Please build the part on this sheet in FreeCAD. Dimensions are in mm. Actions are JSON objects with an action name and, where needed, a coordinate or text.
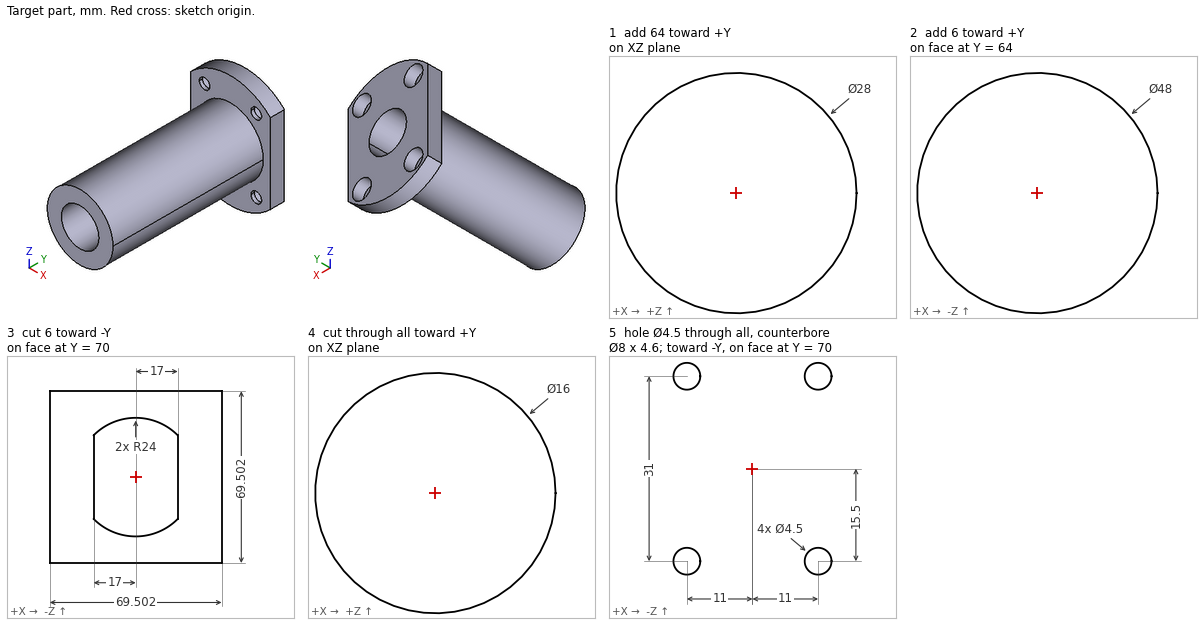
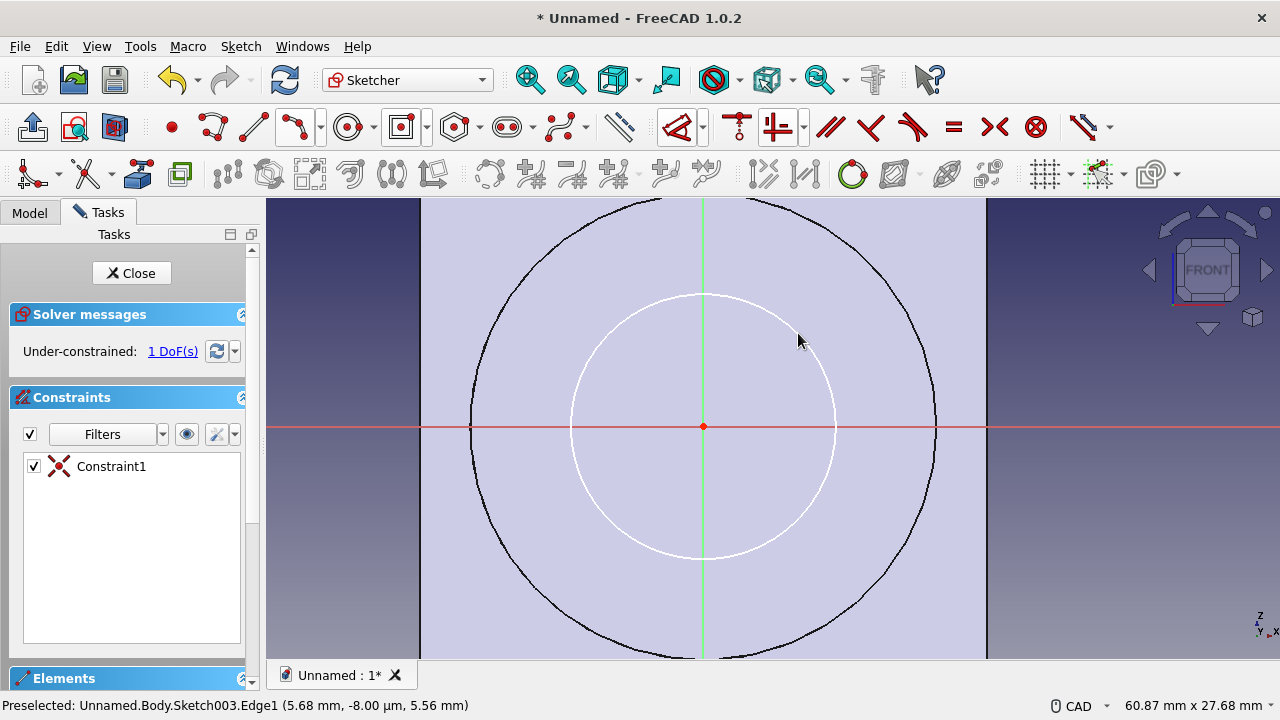
{"action": "left_click", "coordinate": [797, 333]}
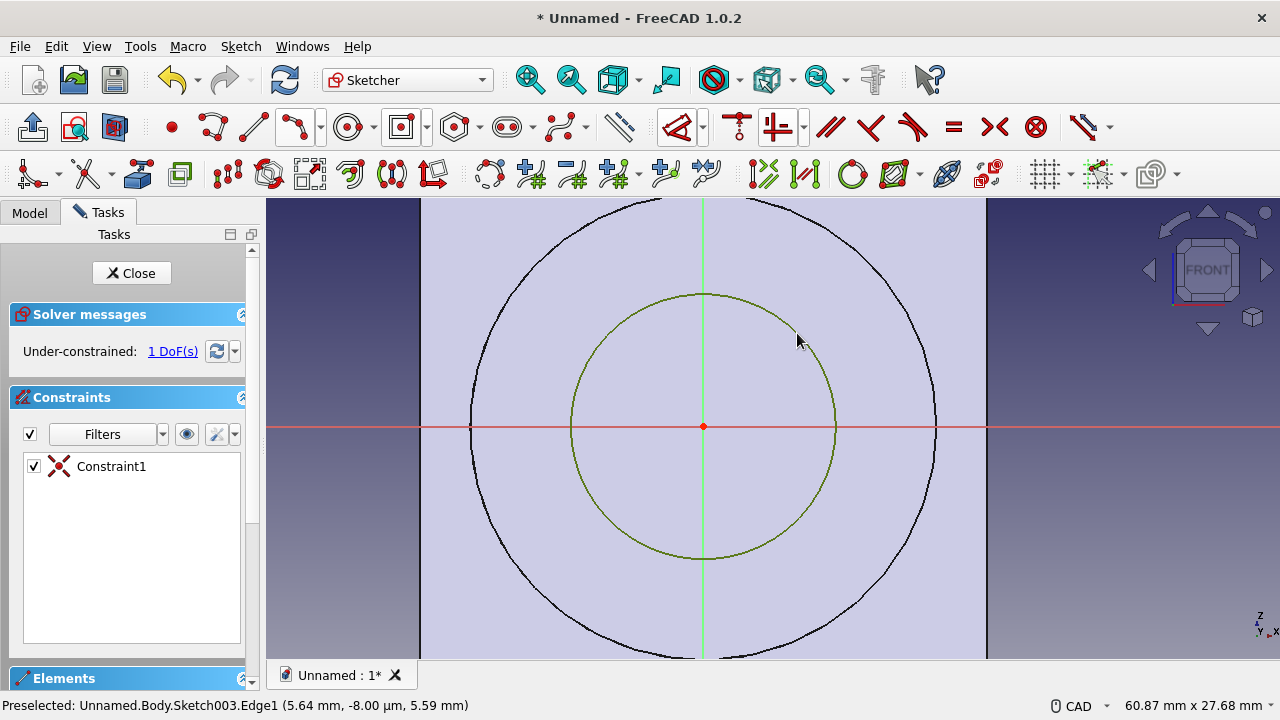
{"action": "left_click", "coordinate": [702, 128]}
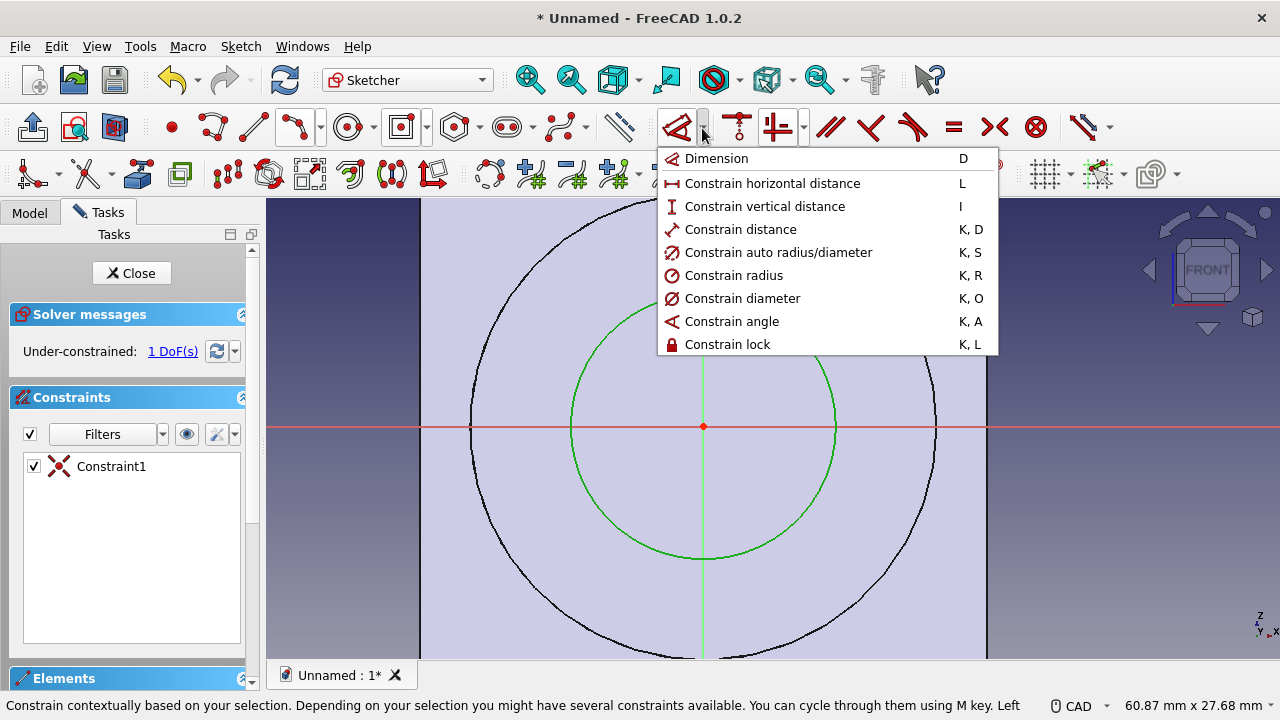
{"action": "left_click", "coordinate": [828, 298]}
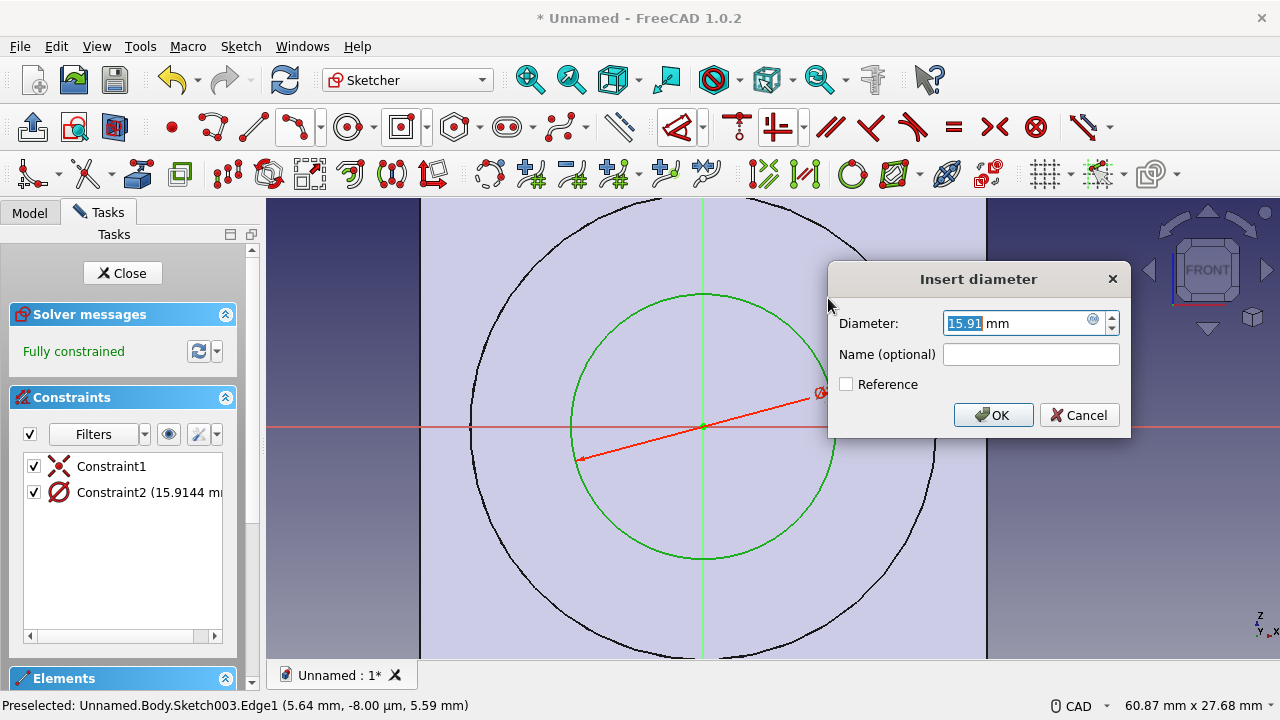
{"action": "type", "text": "16"}
{"action": "key", "text": "Return"}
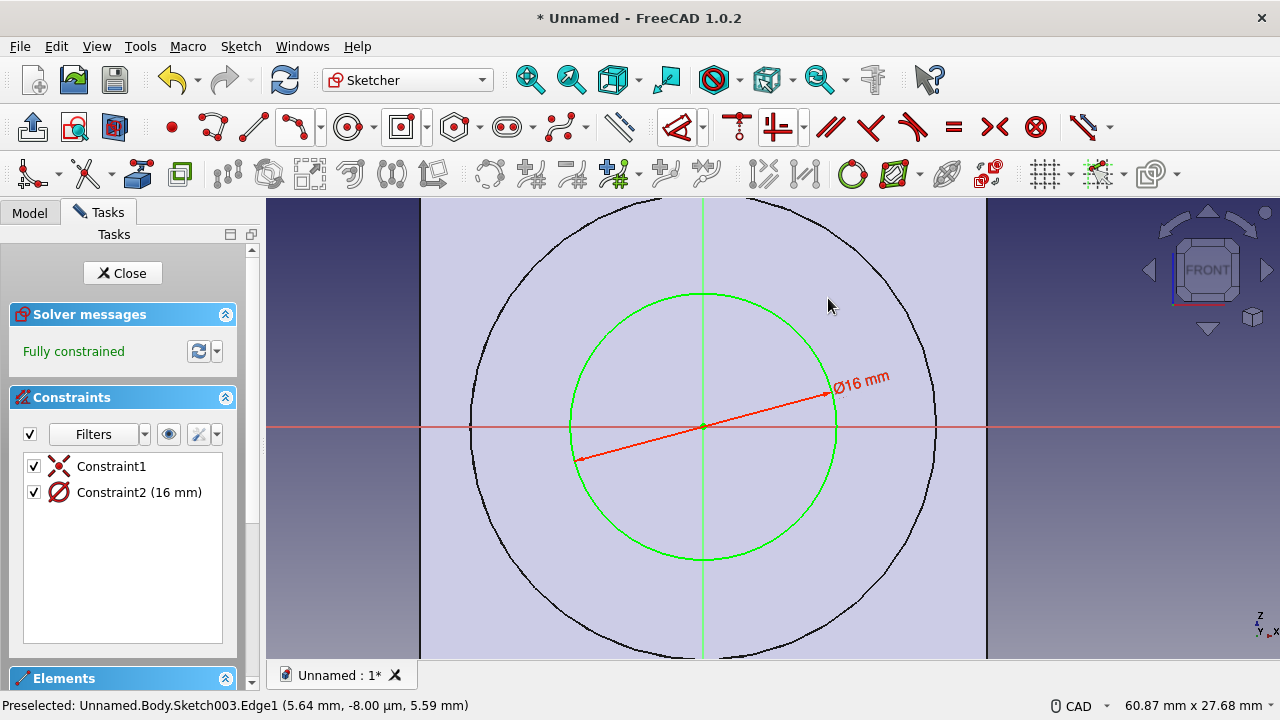
{"action": "left_click", "coordinate": [123, 273]}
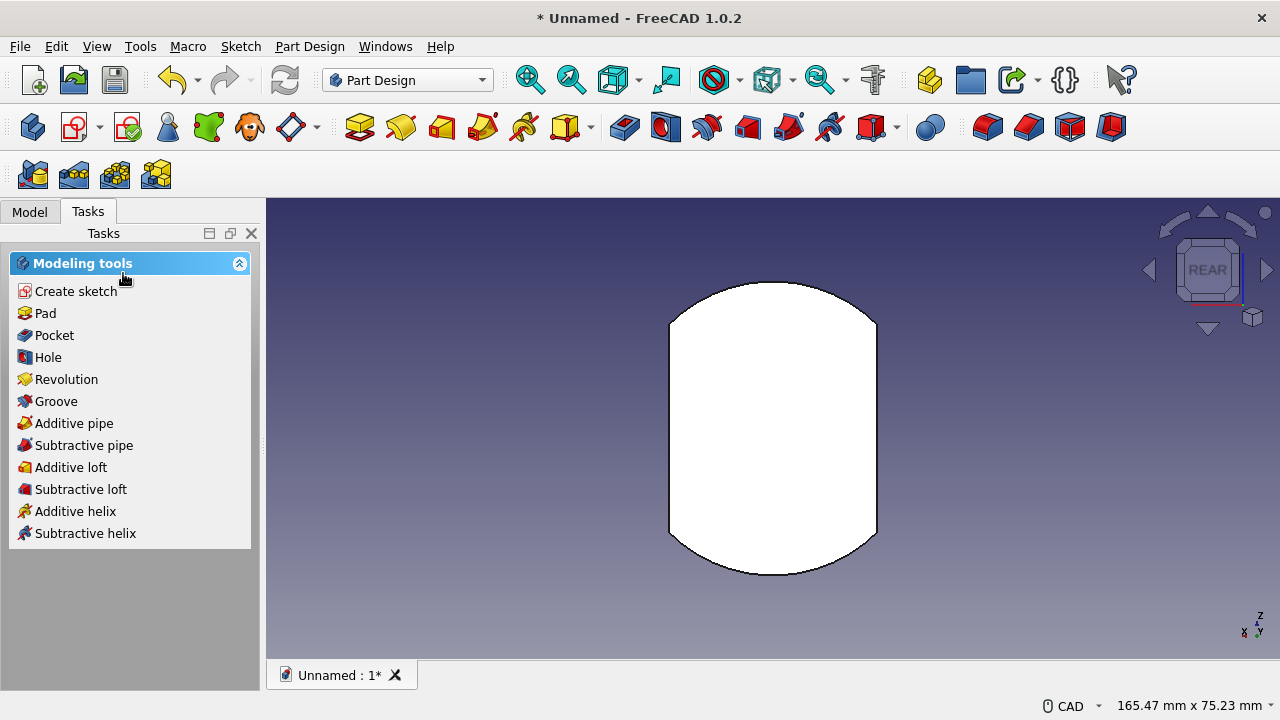
{"action": "left_click", "coordinate": [625, 128]}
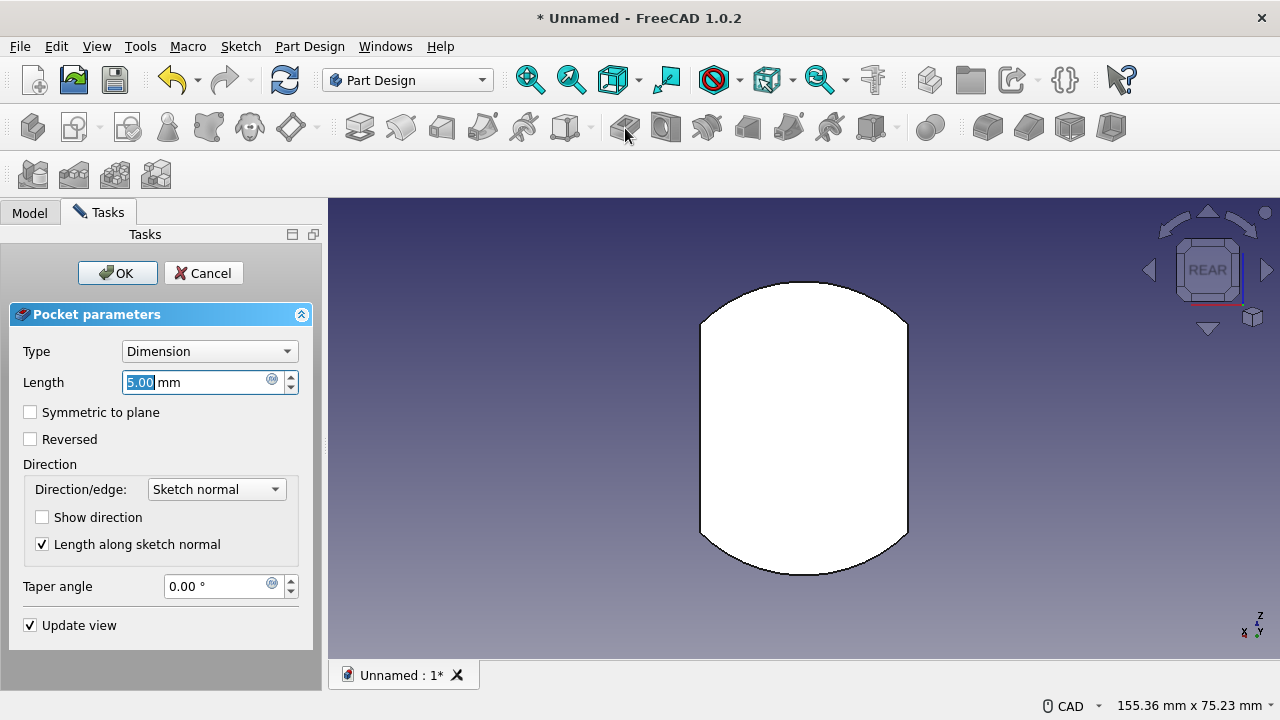
{"action": "left_click", "coordinate": [210, 352]}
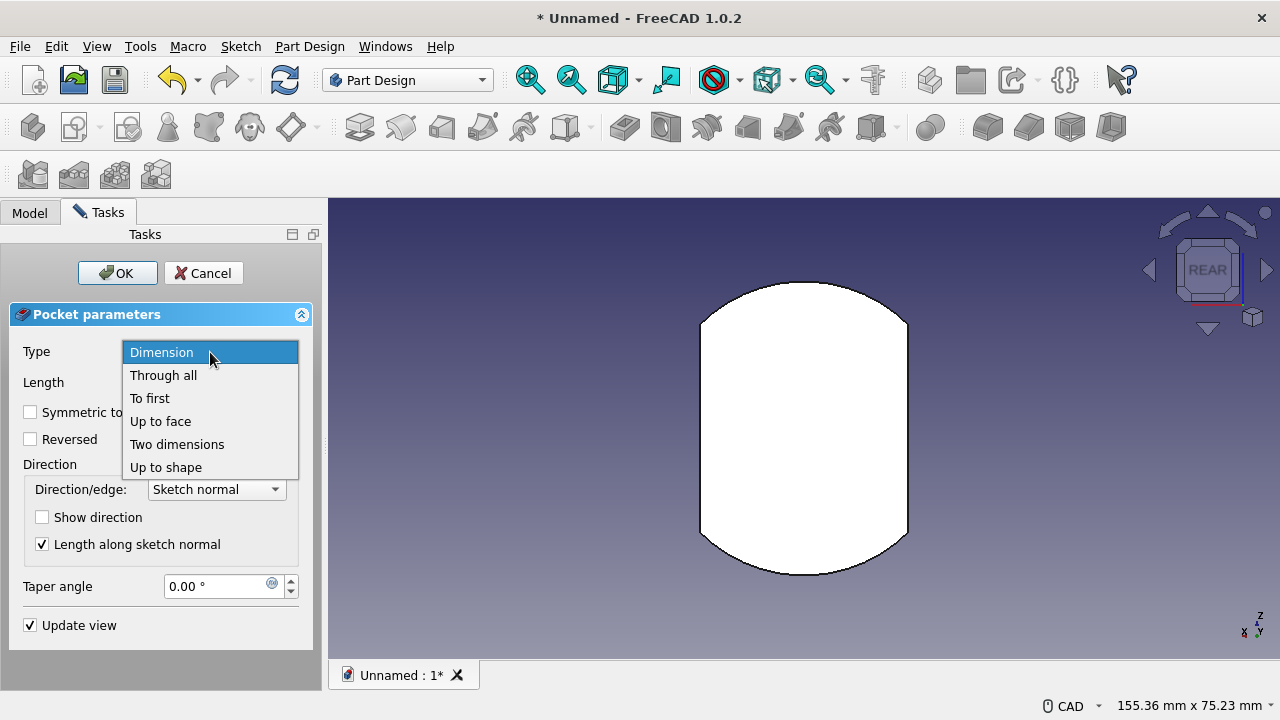
{"action": "left_click", "coordinate": [208, 376]}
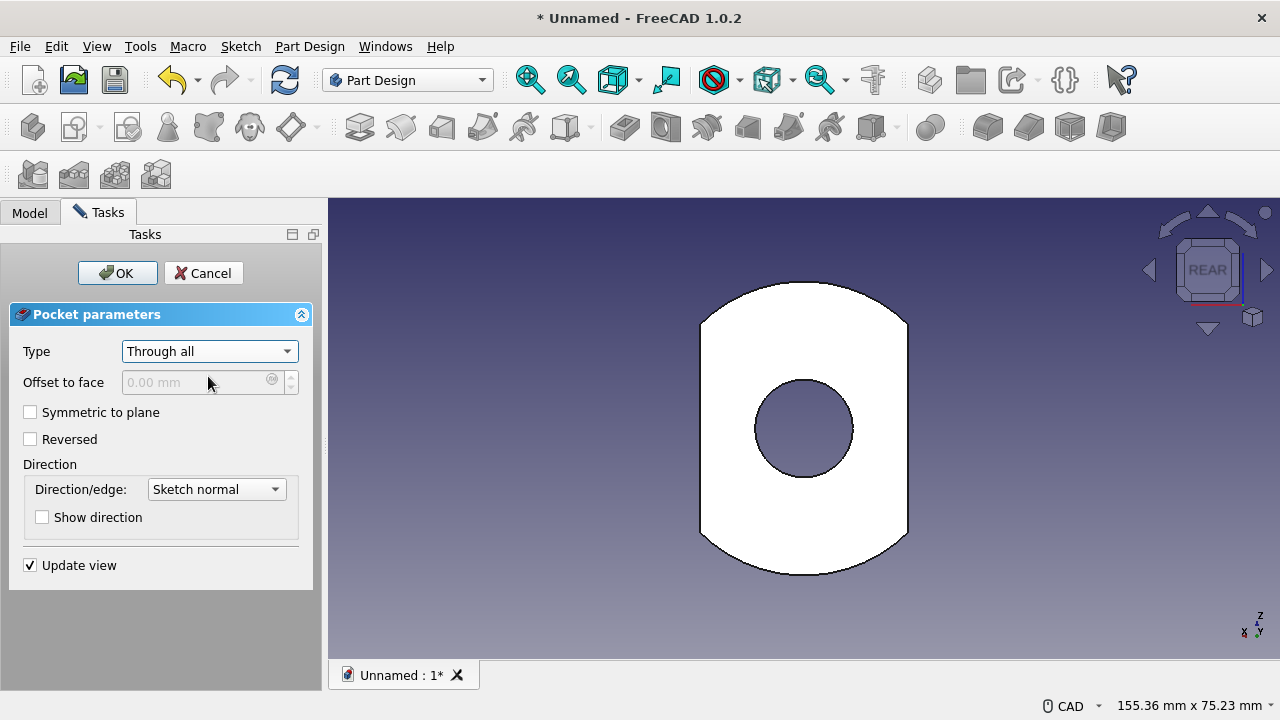
{"action": "left_click", "coordinate": [118, 273]}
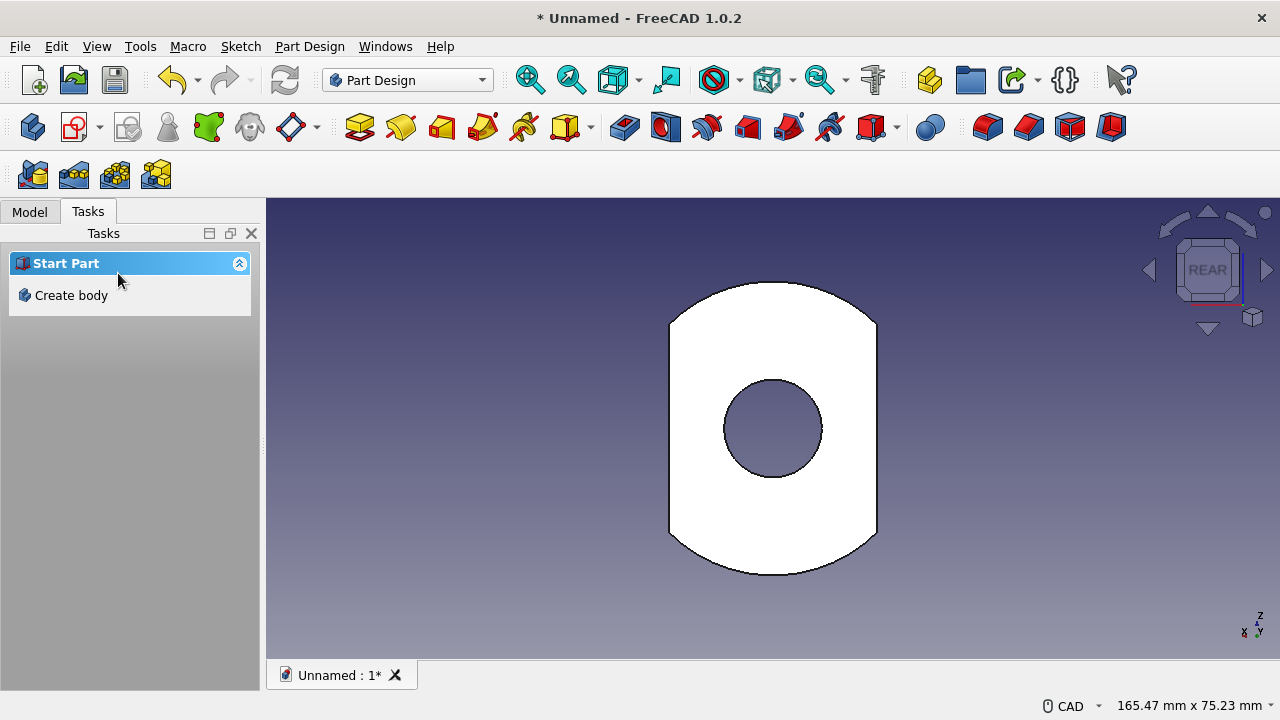
{"action": "left_click", "coordinate": [713, 512]}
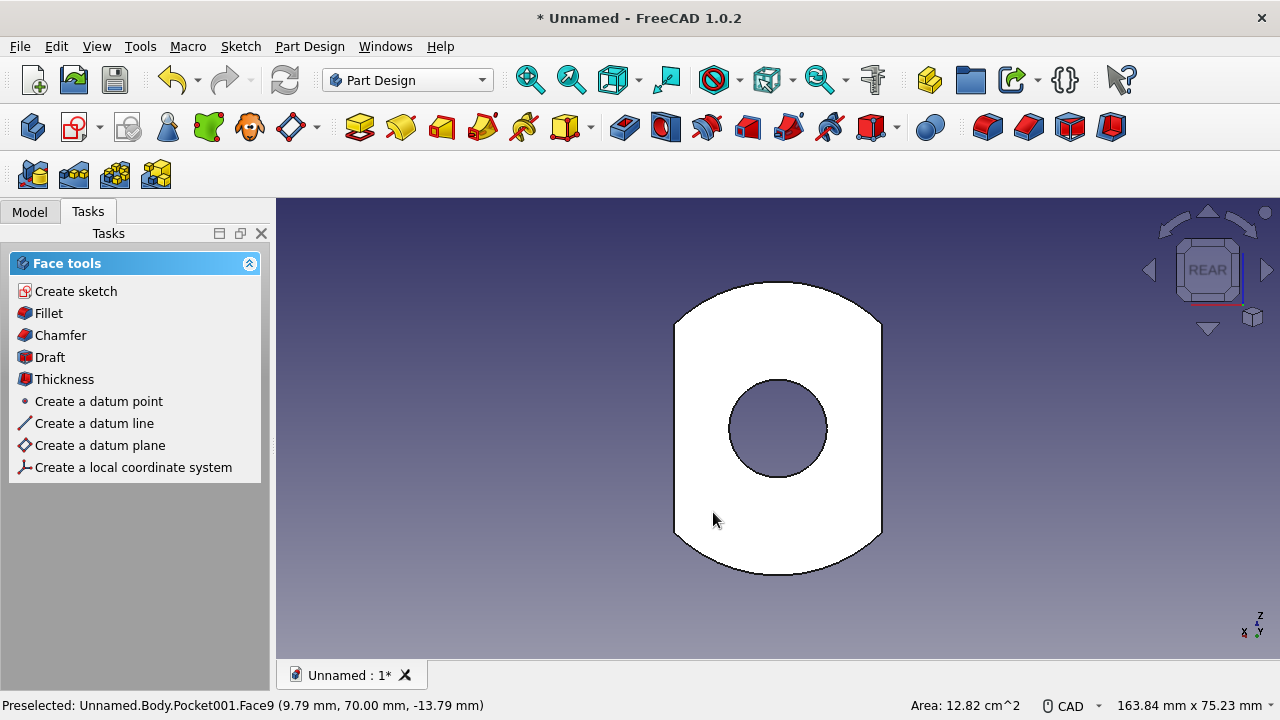
{"action": "left_click", "coordinate": [74, 128]}